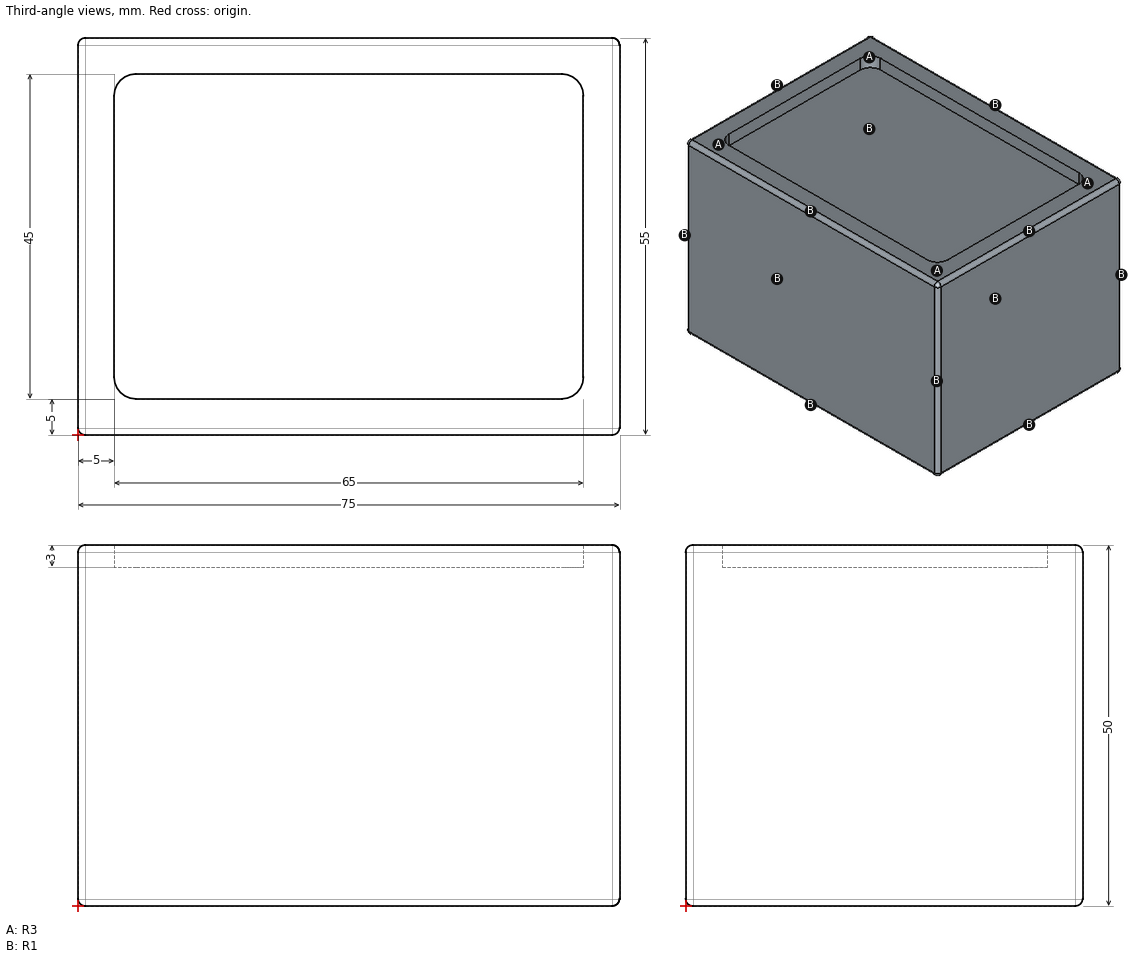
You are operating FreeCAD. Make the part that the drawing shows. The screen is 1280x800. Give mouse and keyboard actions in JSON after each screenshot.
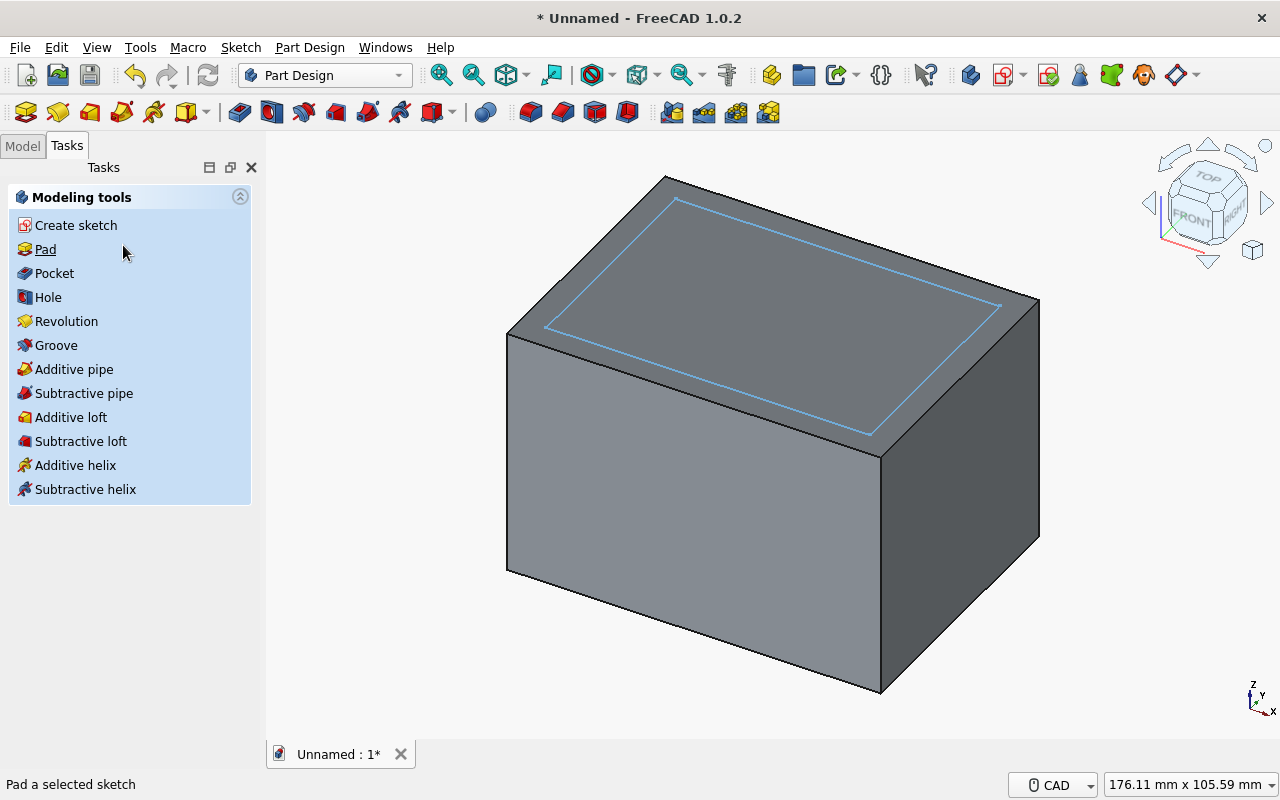
{"action": "left_click", "coordinate": [240, 112]}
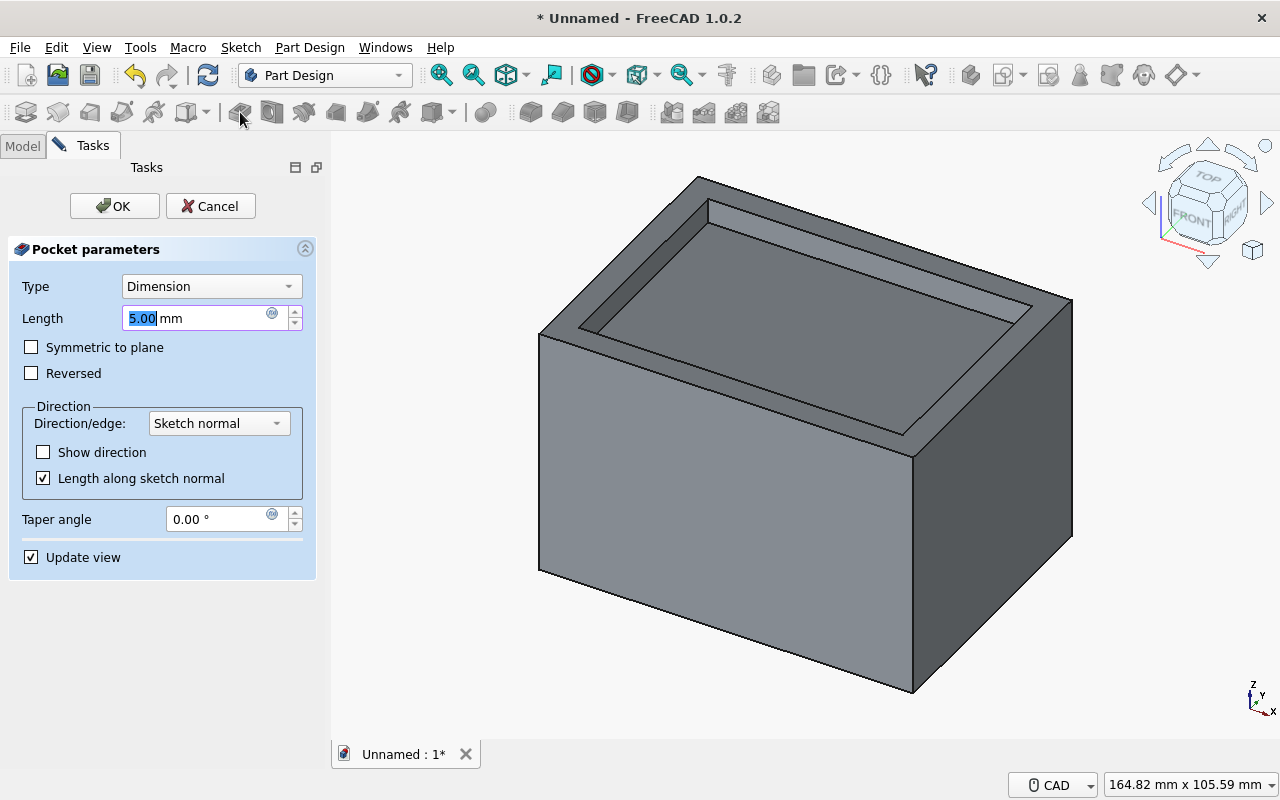
{"action": "type", "text": "3"}
{"action": "key", "text": "Tab"}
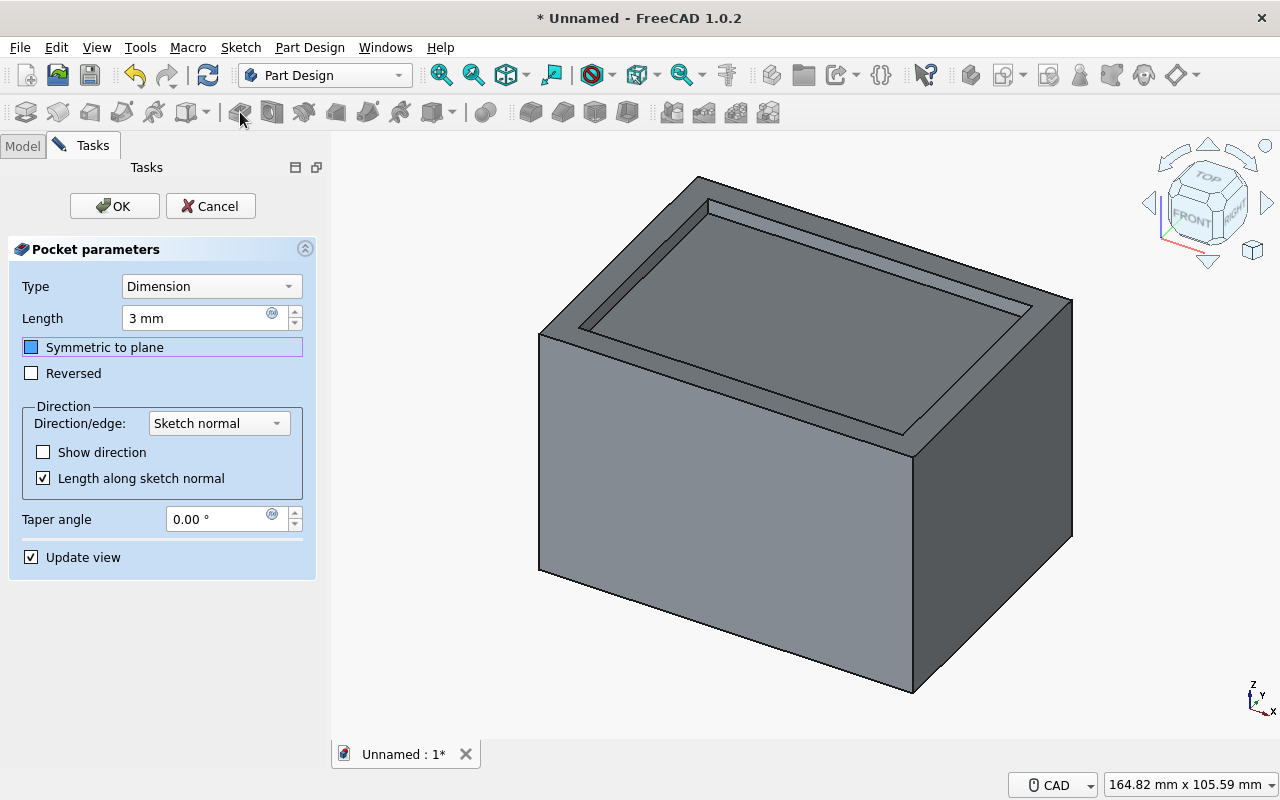
{"action": "left_click", "coordinate": [115, 206]}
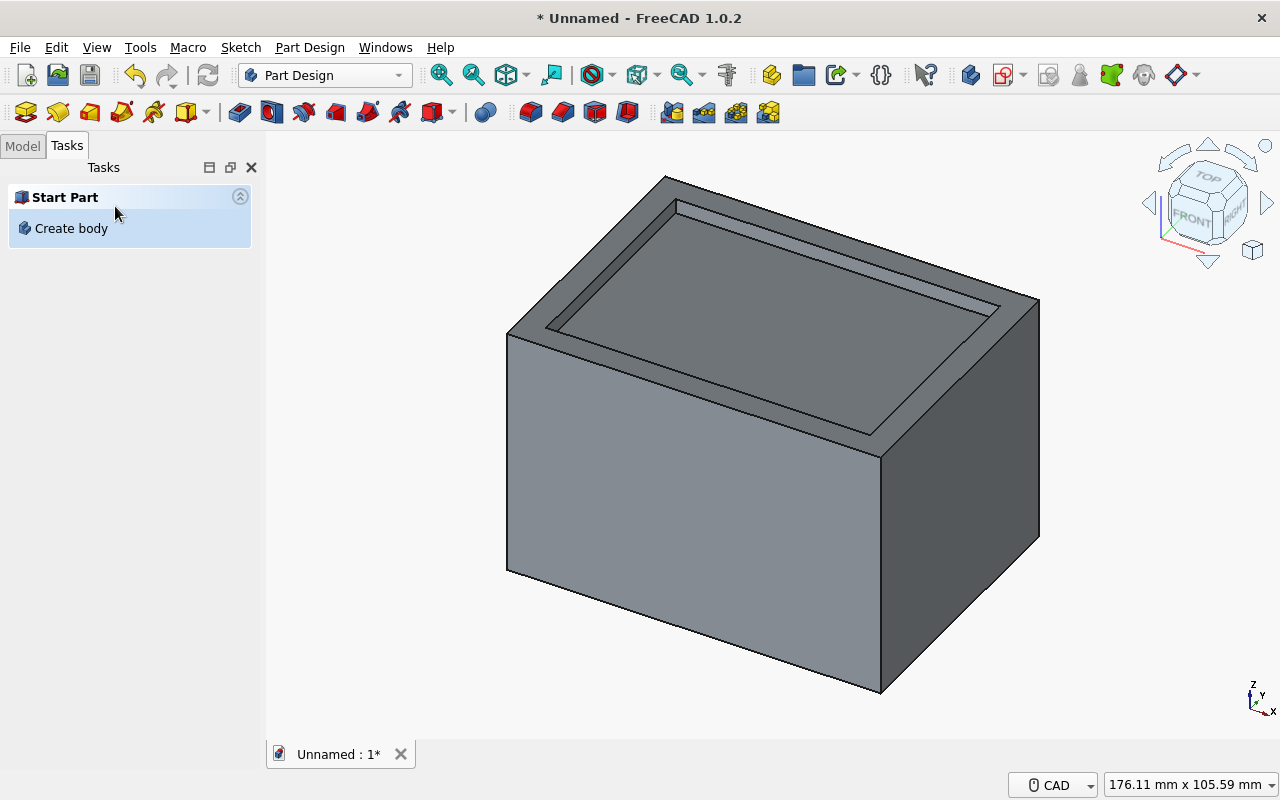
{"action": "scroll", "coordinate": [546, 334], "scroll_direction": "up", "scroll_amount": 5}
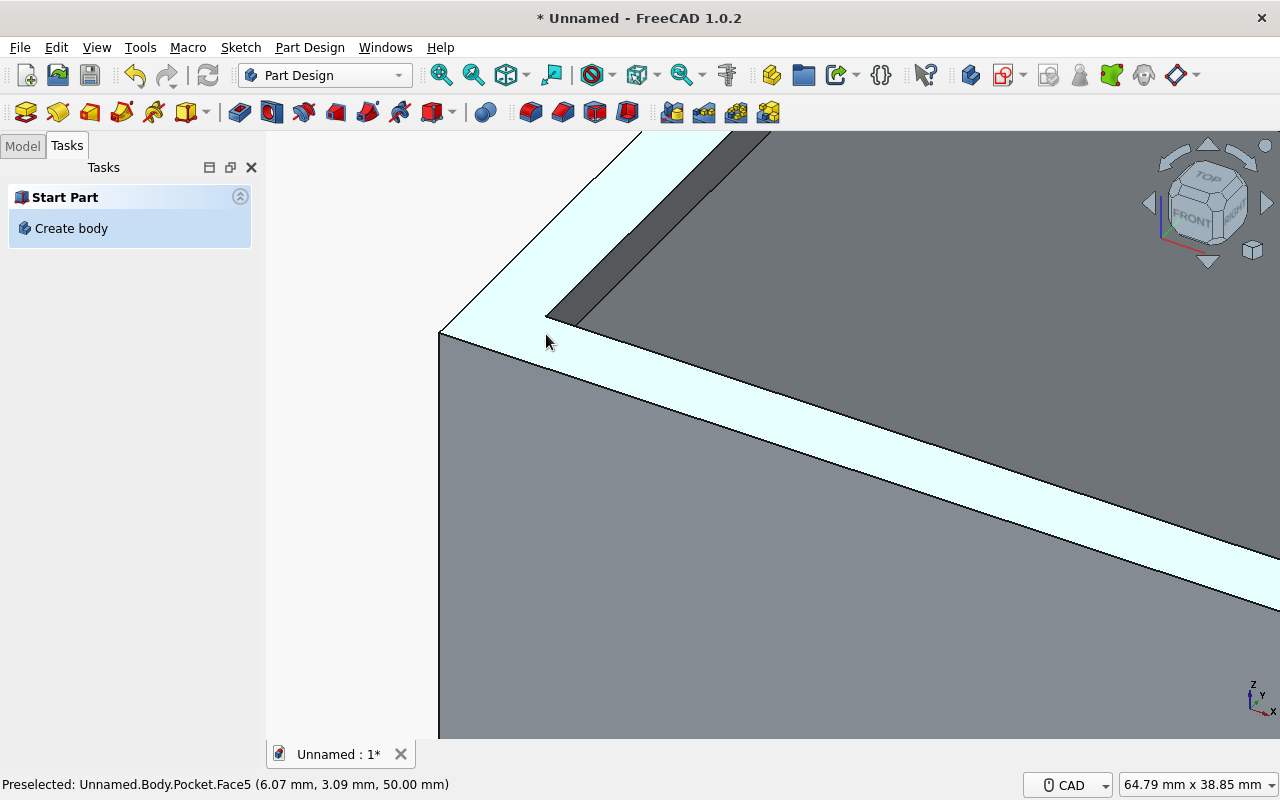
{"action": "left_click", "coordinate": [442, 76]}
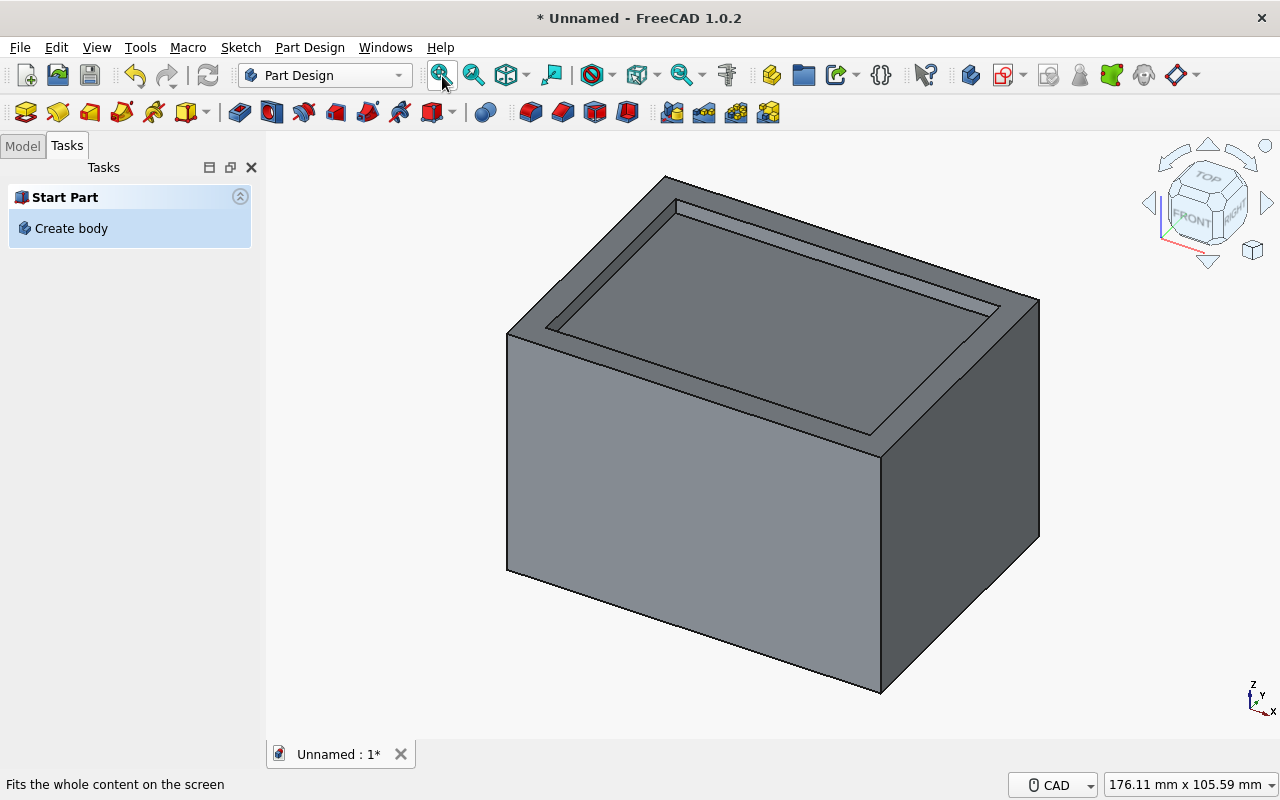
{"action": "key", "text": "0"}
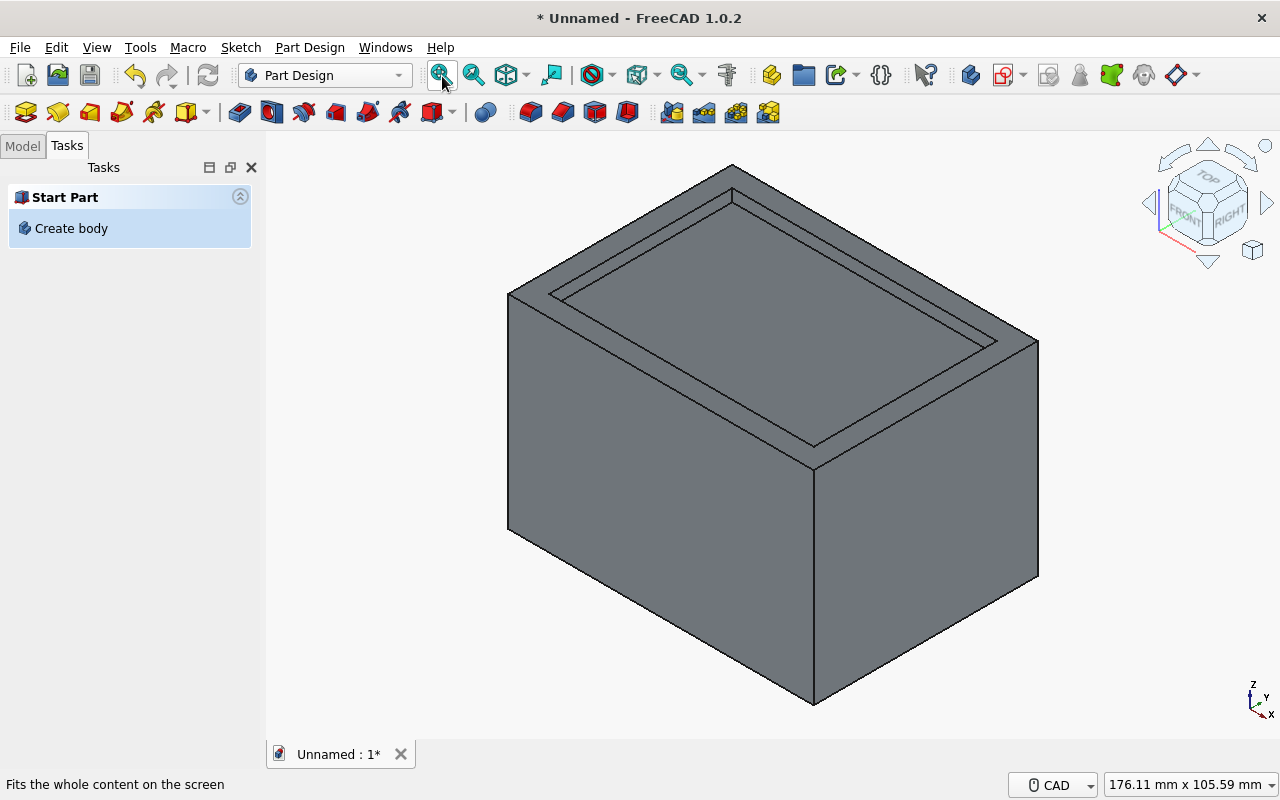
{"action": "scroll", "coordinate": [549, 300], "scroll_direction": "up", "scroll_amount": 5}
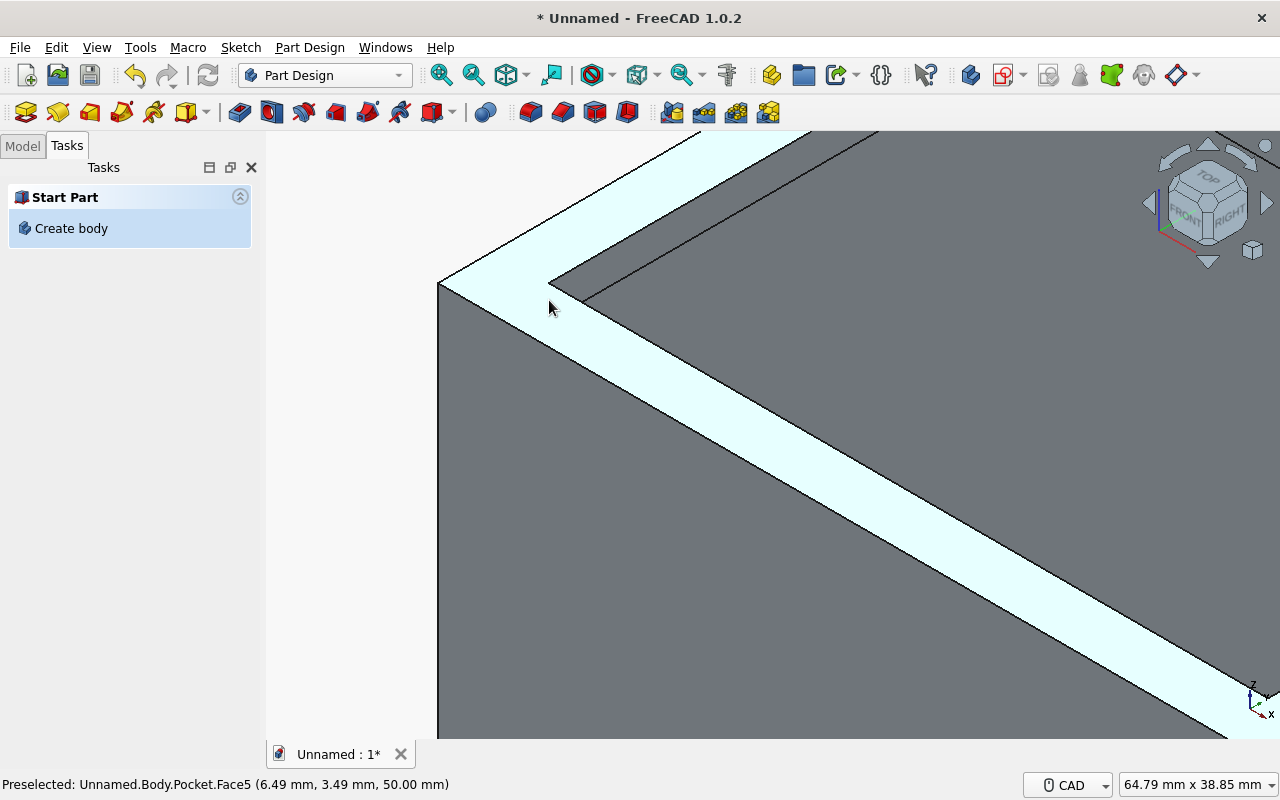
{"action": "left_click", "coordinate": [442, 76]}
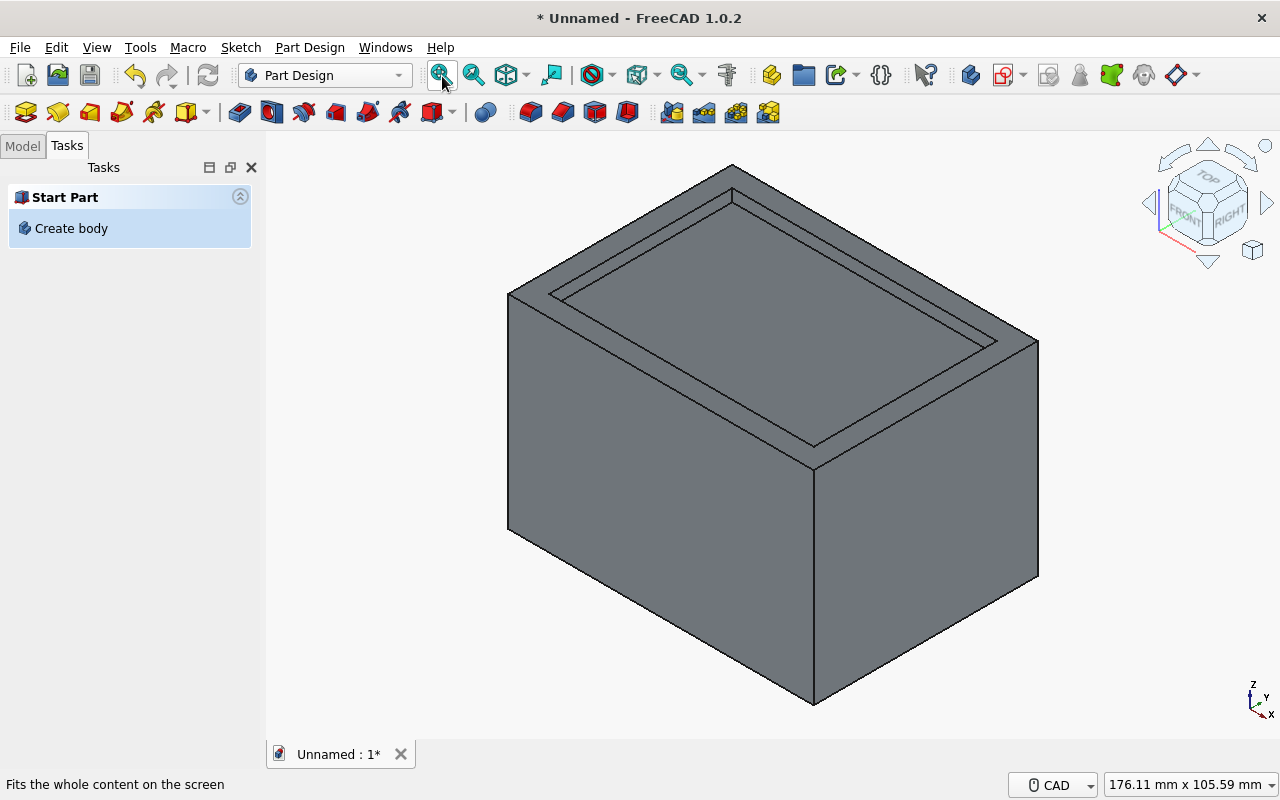
{"action": "key", "text": "2"}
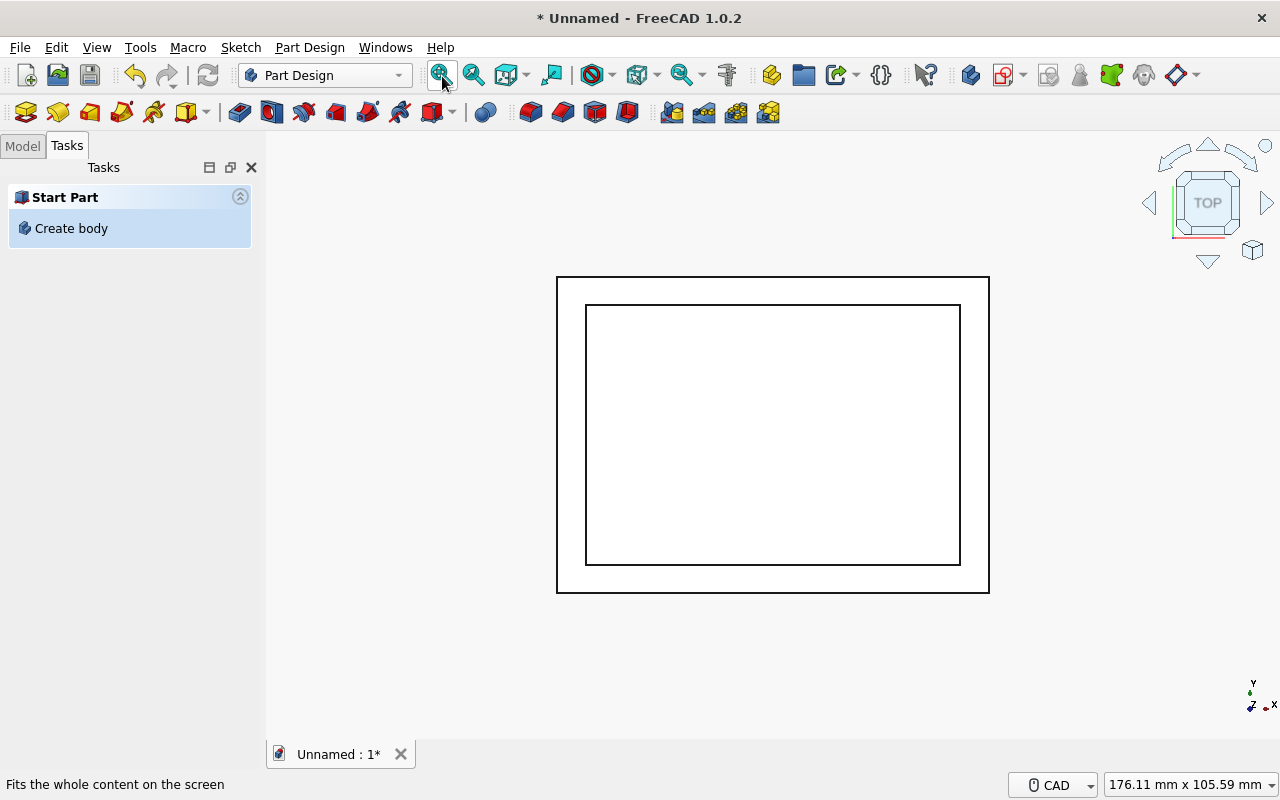
{"action": "scroll", "coordinate": [586, 564], "scroll_direction": "up", "scroll_amount": 5}